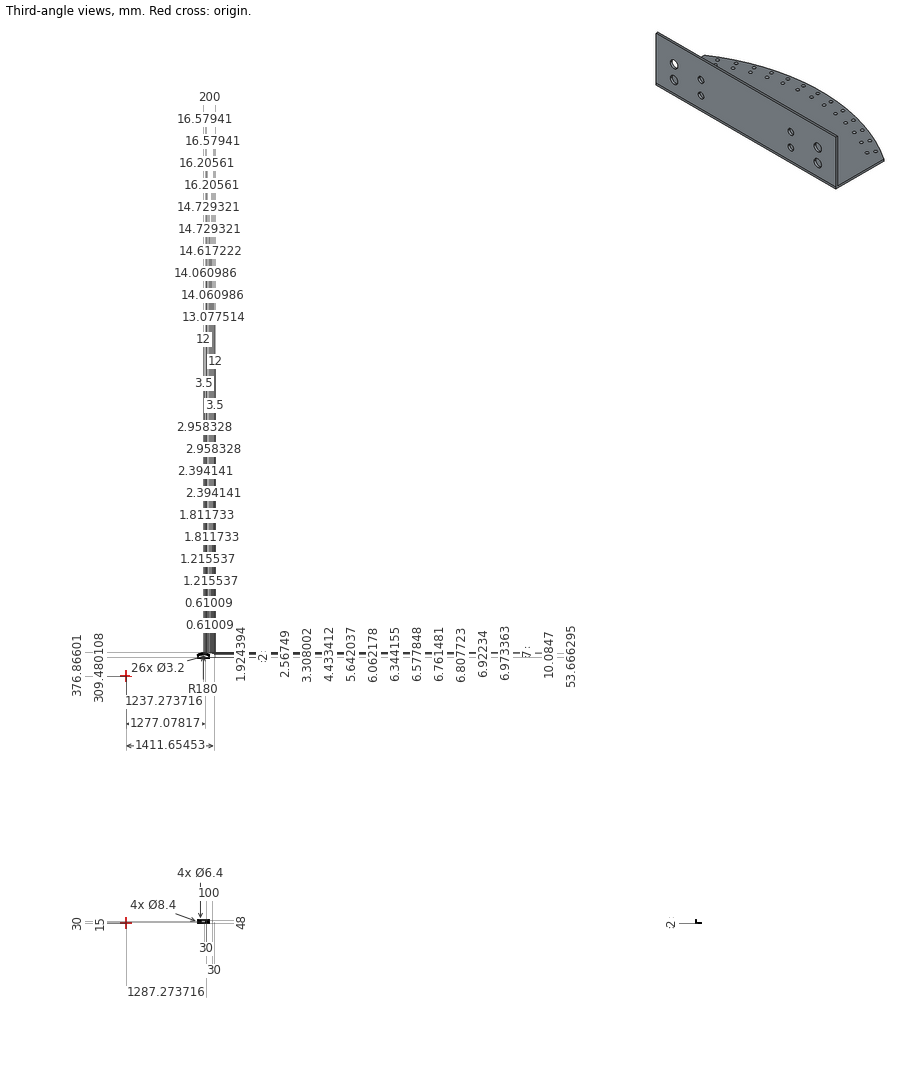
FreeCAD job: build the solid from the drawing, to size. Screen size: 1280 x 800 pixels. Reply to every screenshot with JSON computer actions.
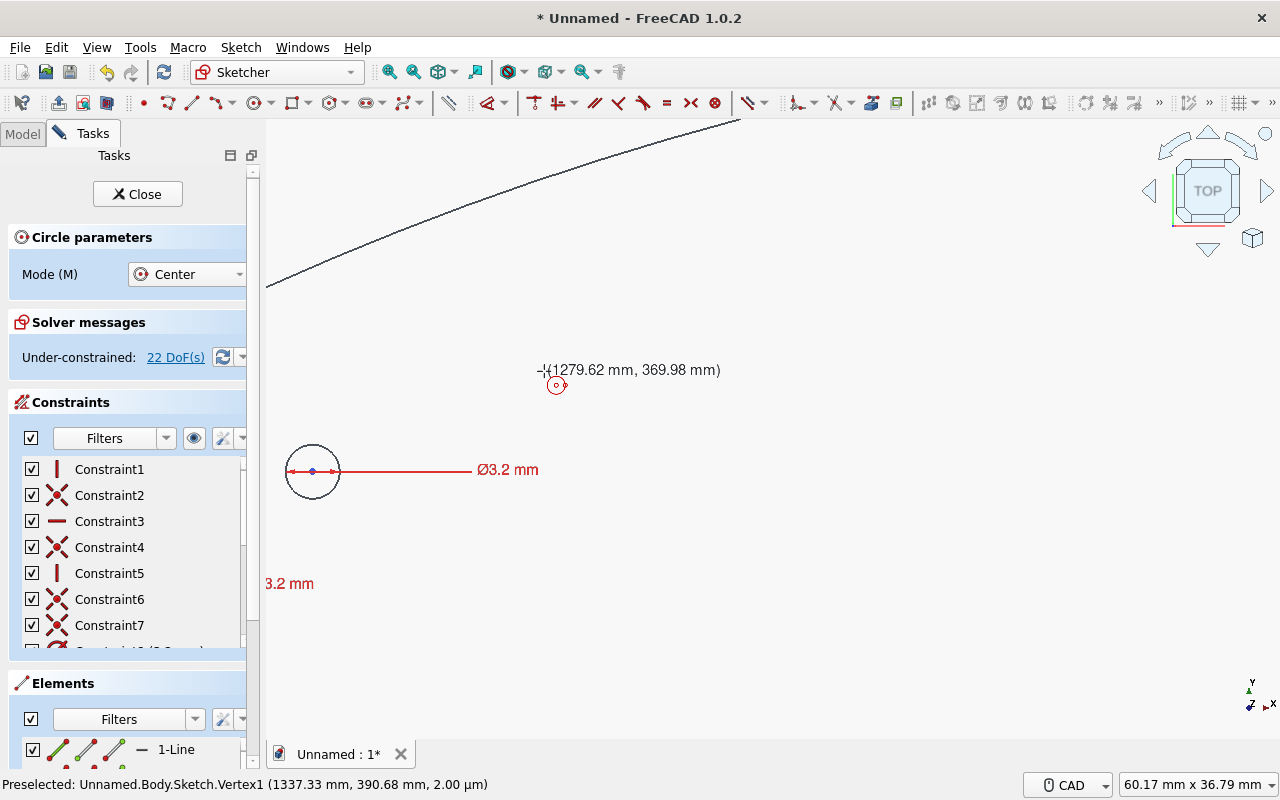
{"action": "scroll", "coordinate": [544, 371], "scroll_direction": "down", "scroll_amount": 9}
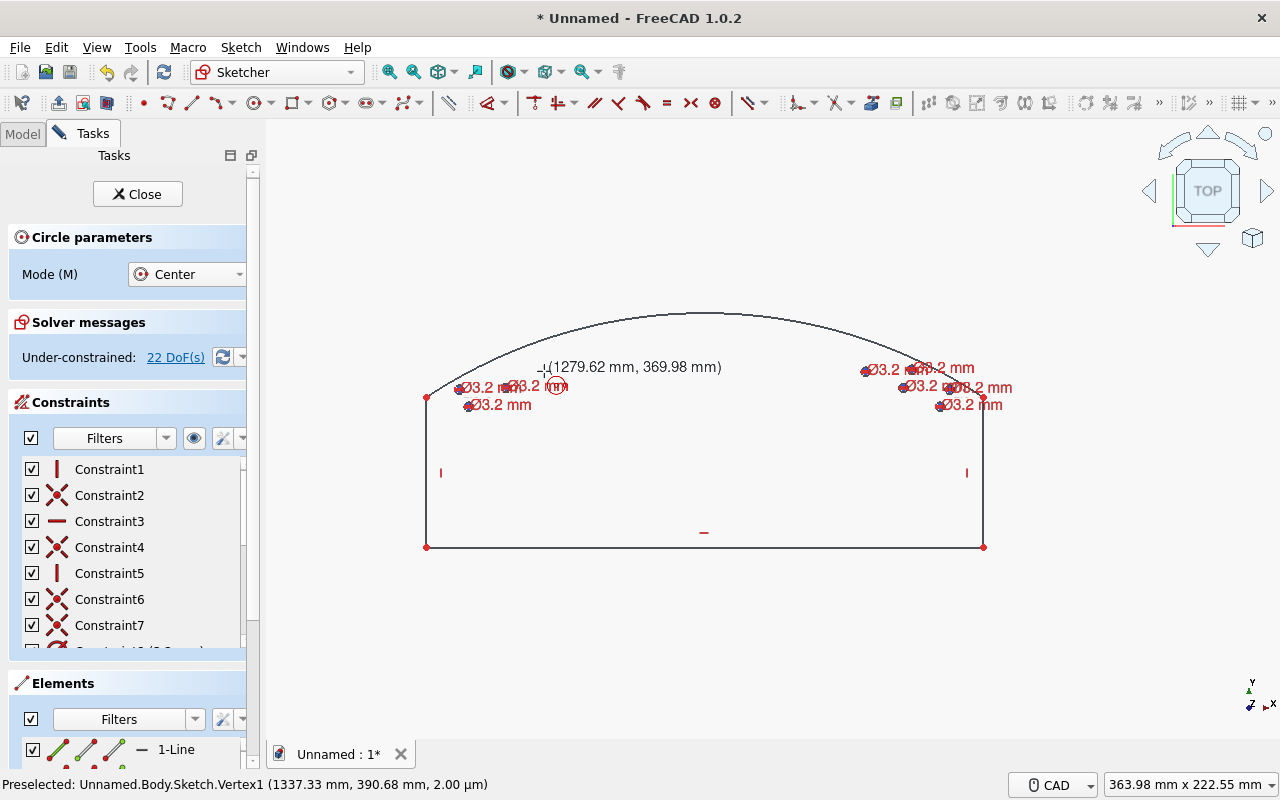
{"action": "left_click", "coordinate": [544, 371]}
{"action": "mouse_move", "coordinate": [547, 368]}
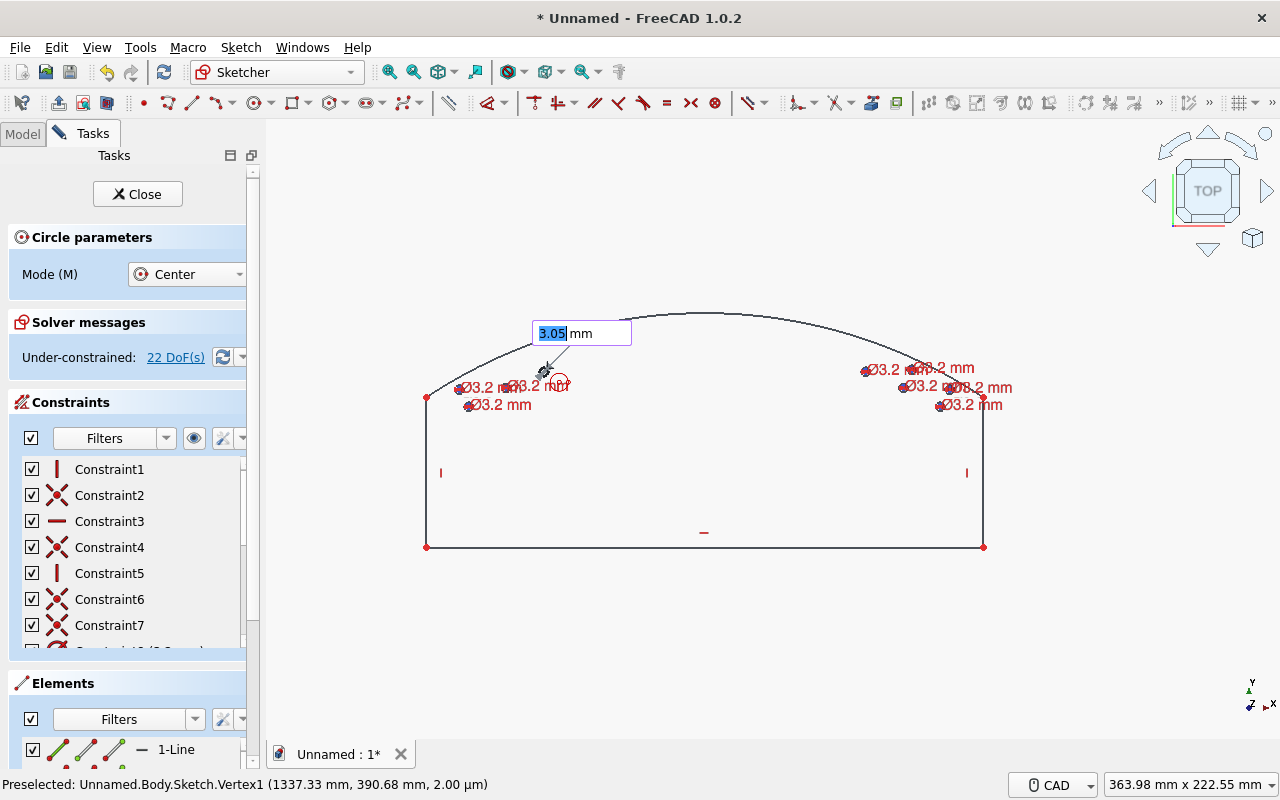
{"action": "type", "text": "3.2"}
{"action": "key", "text": "Return"}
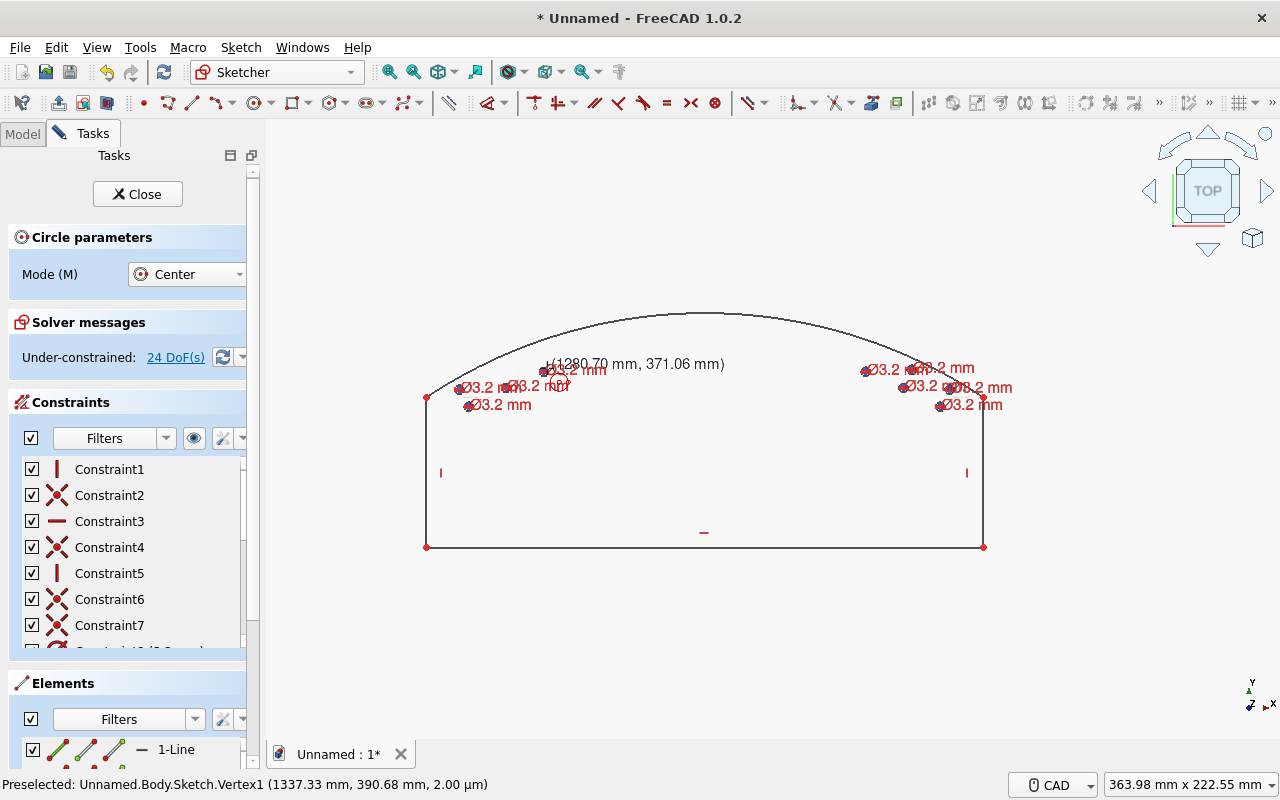
{"action": "scroll", "coordinate": [497, 369], "scroll_direction": "up", "scroll_amount": 9}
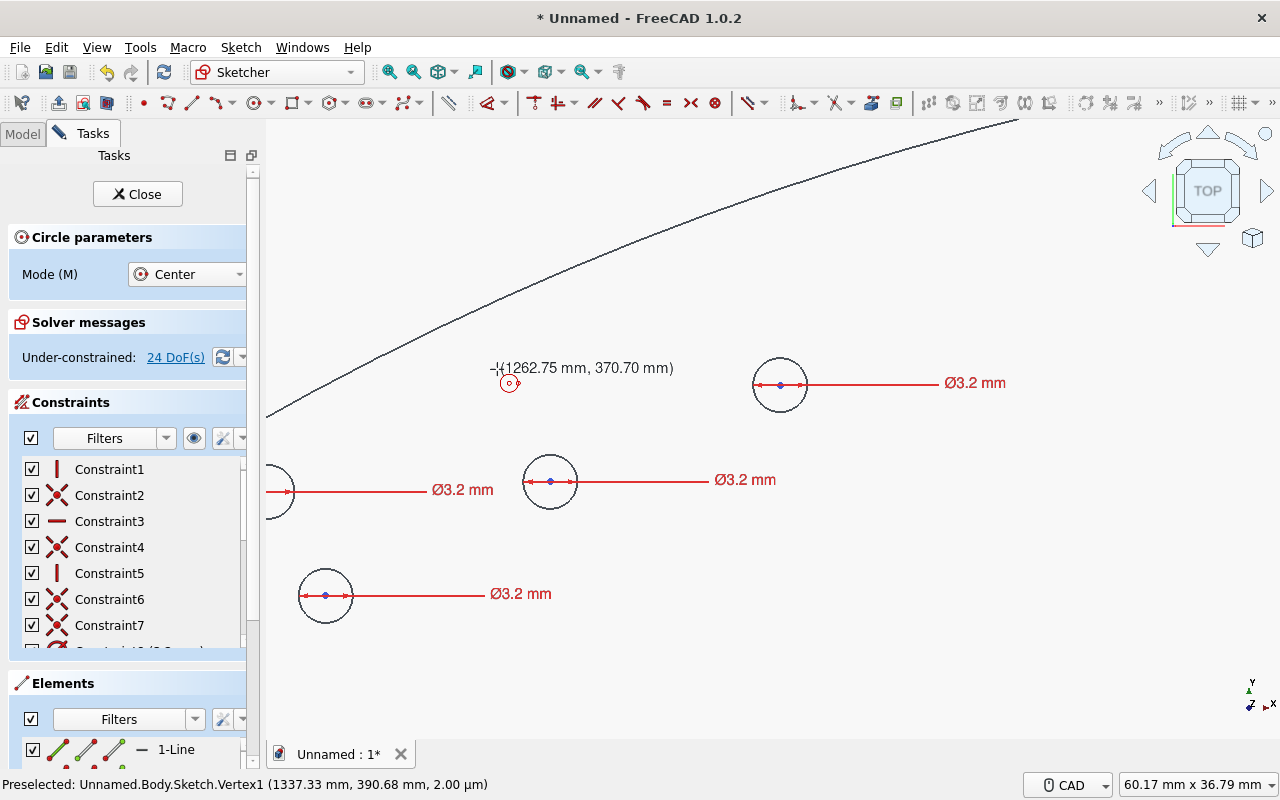
{"action": "scroll", "coordinate": [497, 369], "scroll_direction": "down", "scroll_amount": 9}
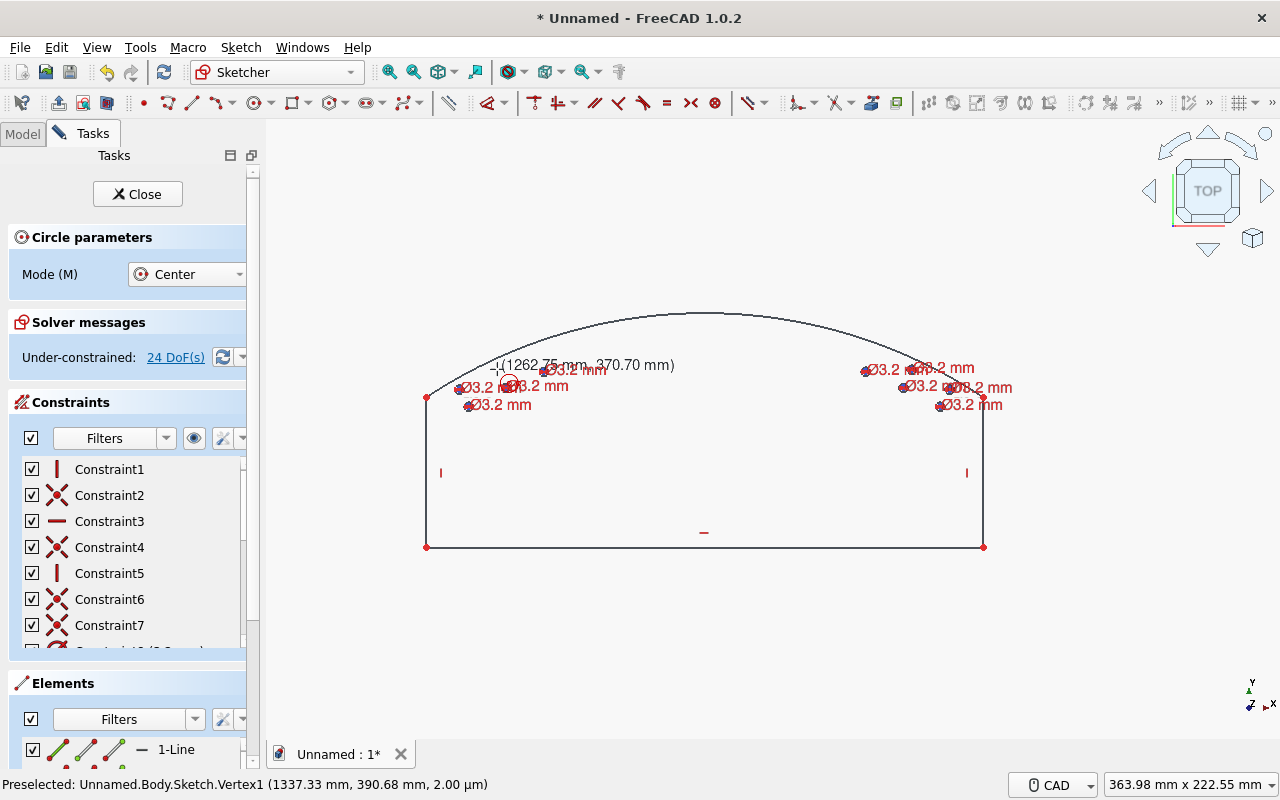
{"action": "scroll", "coordinate": [497, 369], "scroll_direction": "up", "scroll_amount": 2}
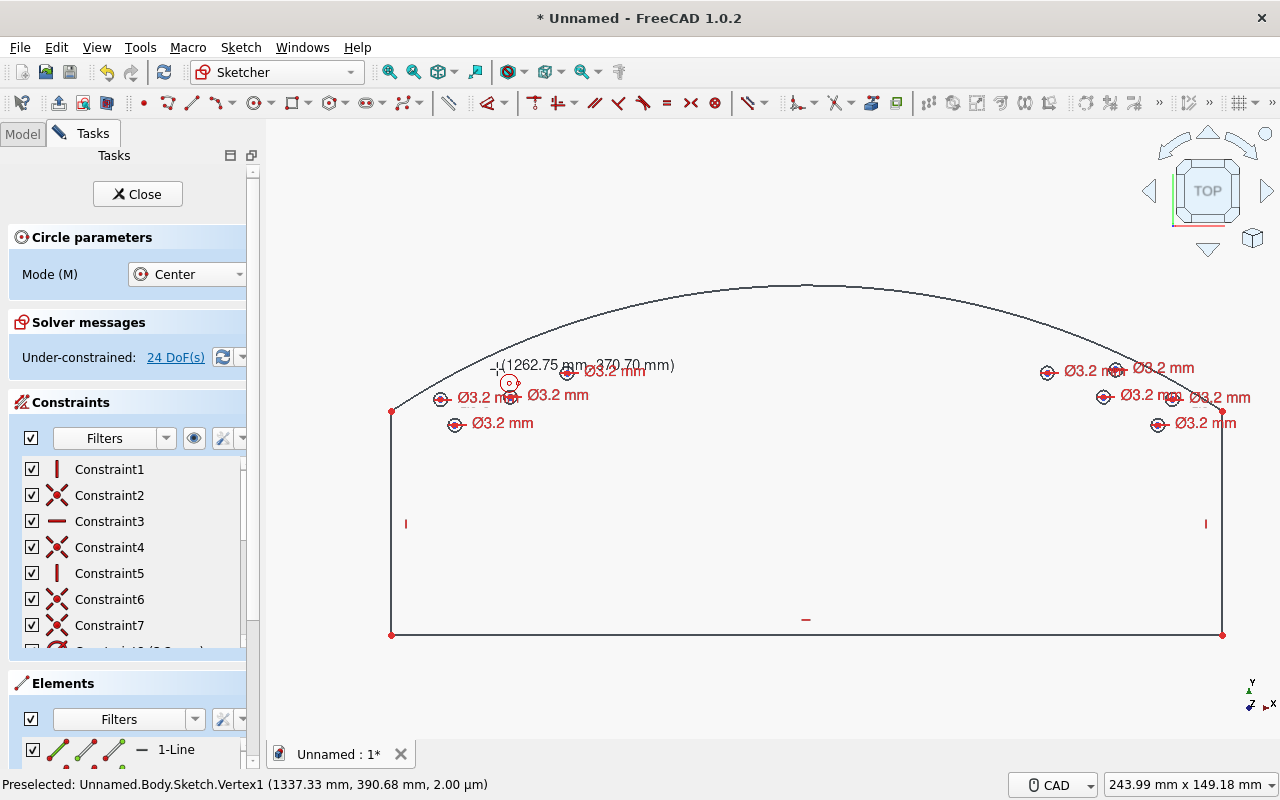
{"action": "left_click", "coordinate": [497, 369]}
{"action": "mouse_move", "coordinate": [502, 364]}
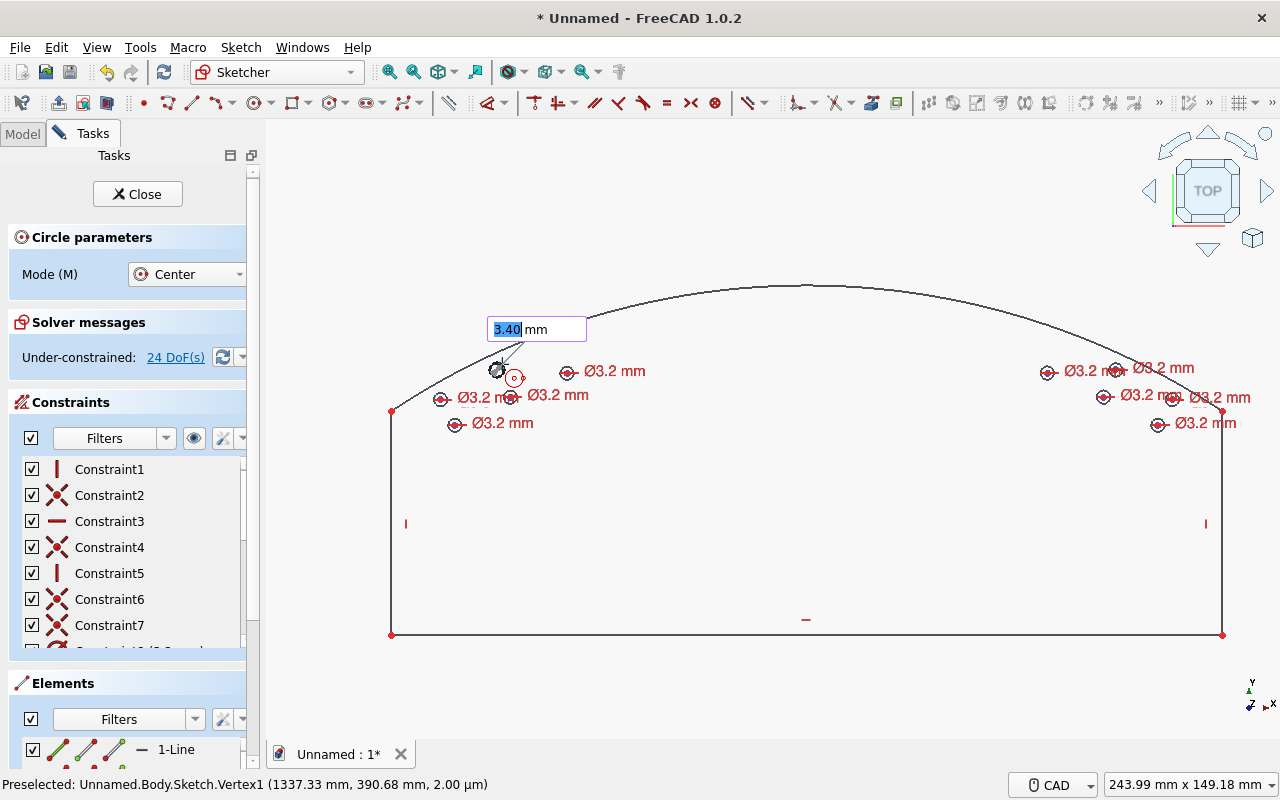
{"action": "type", "text": "3.2"}
{"action": "key", "text": "Return"}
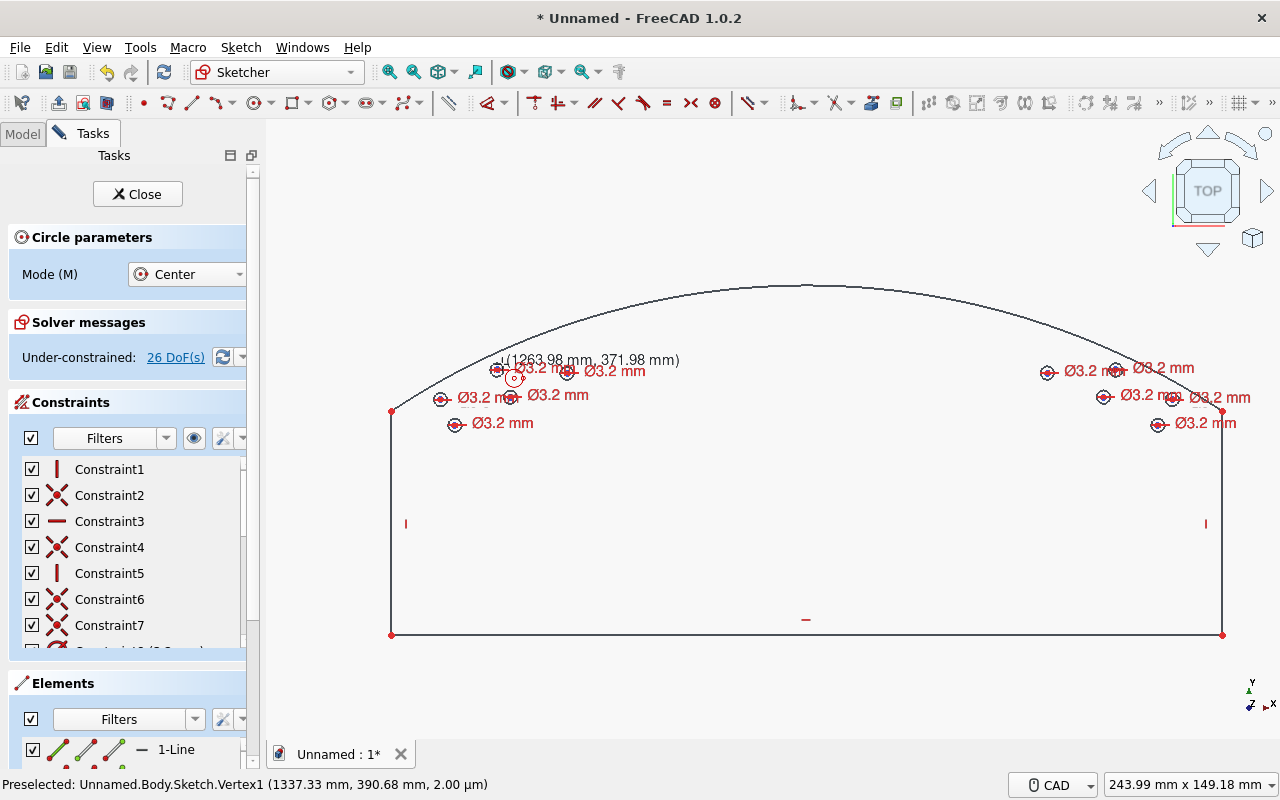
{"action": "scroll", "coordinate": [1057, 345], "scroll_direction": "up", "scroll_amount": 7}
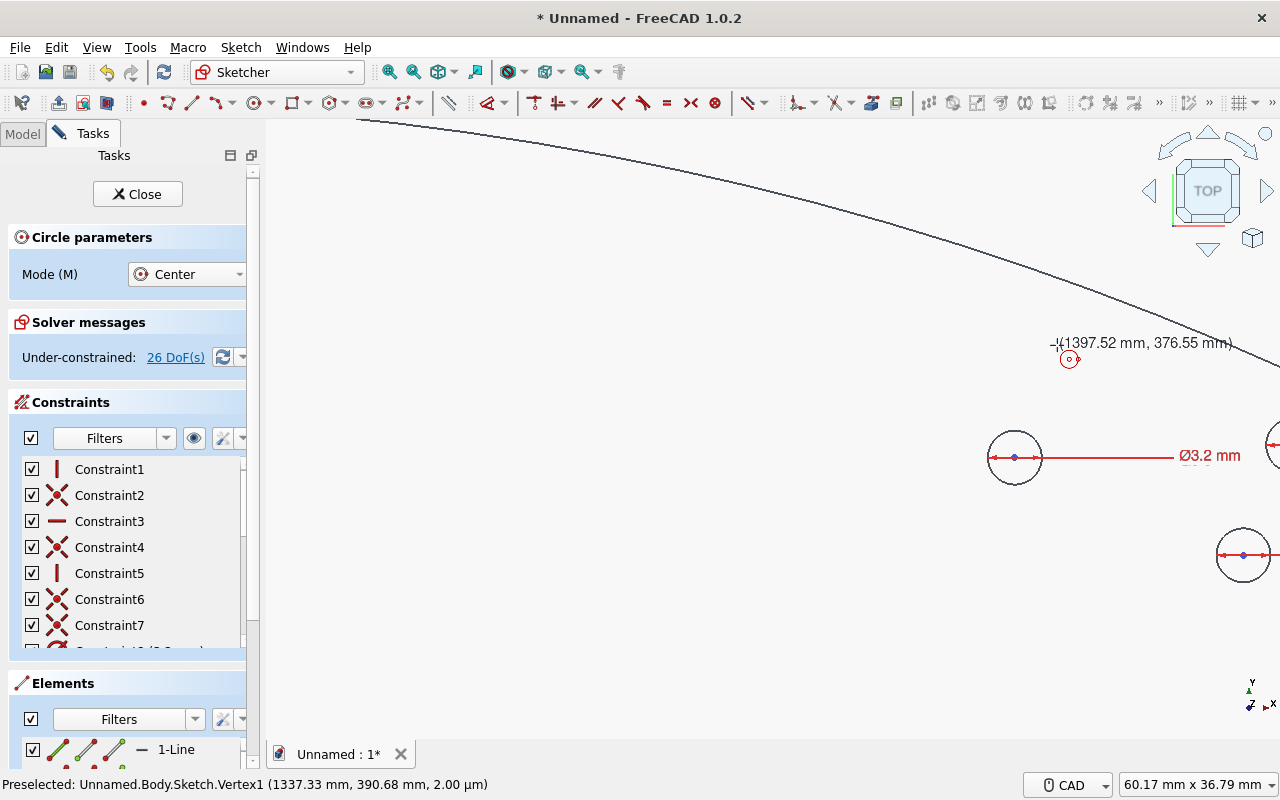
{"action": "scroll", "coordinate": [836, 355], "scroll_direction": "down", "scroll_amount": 9}